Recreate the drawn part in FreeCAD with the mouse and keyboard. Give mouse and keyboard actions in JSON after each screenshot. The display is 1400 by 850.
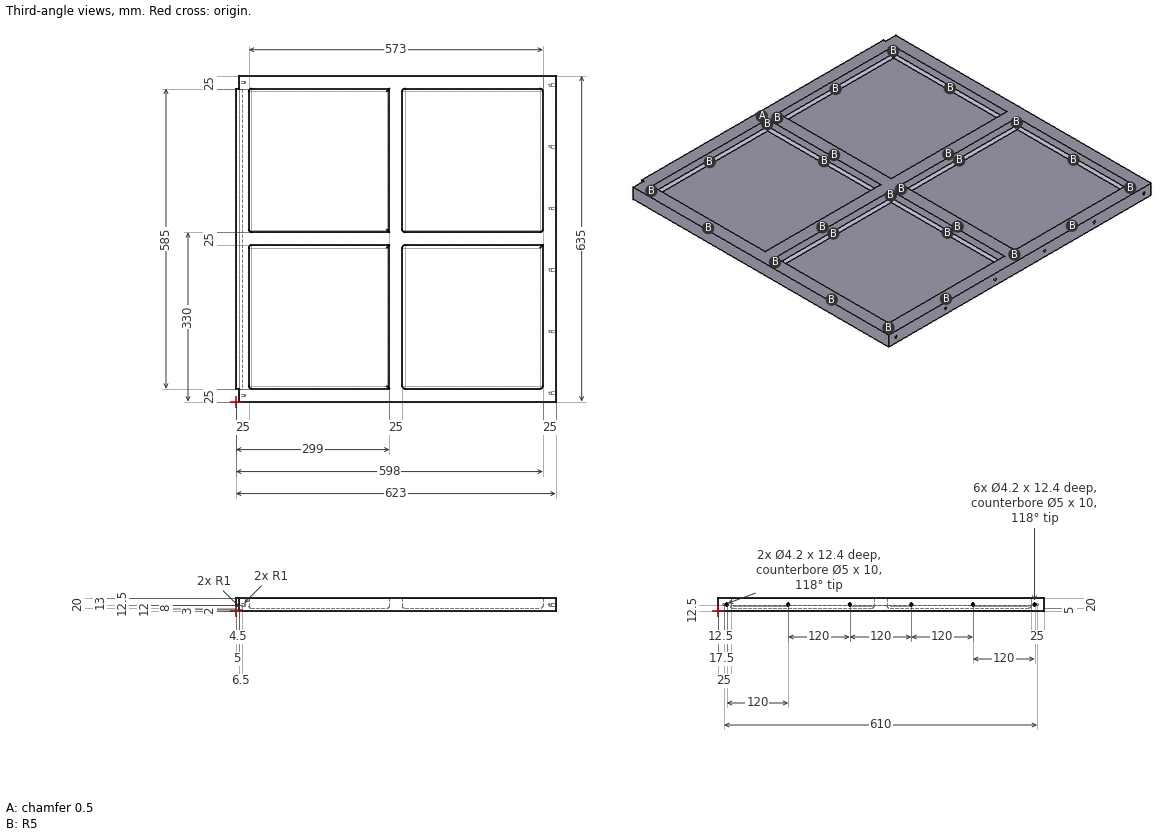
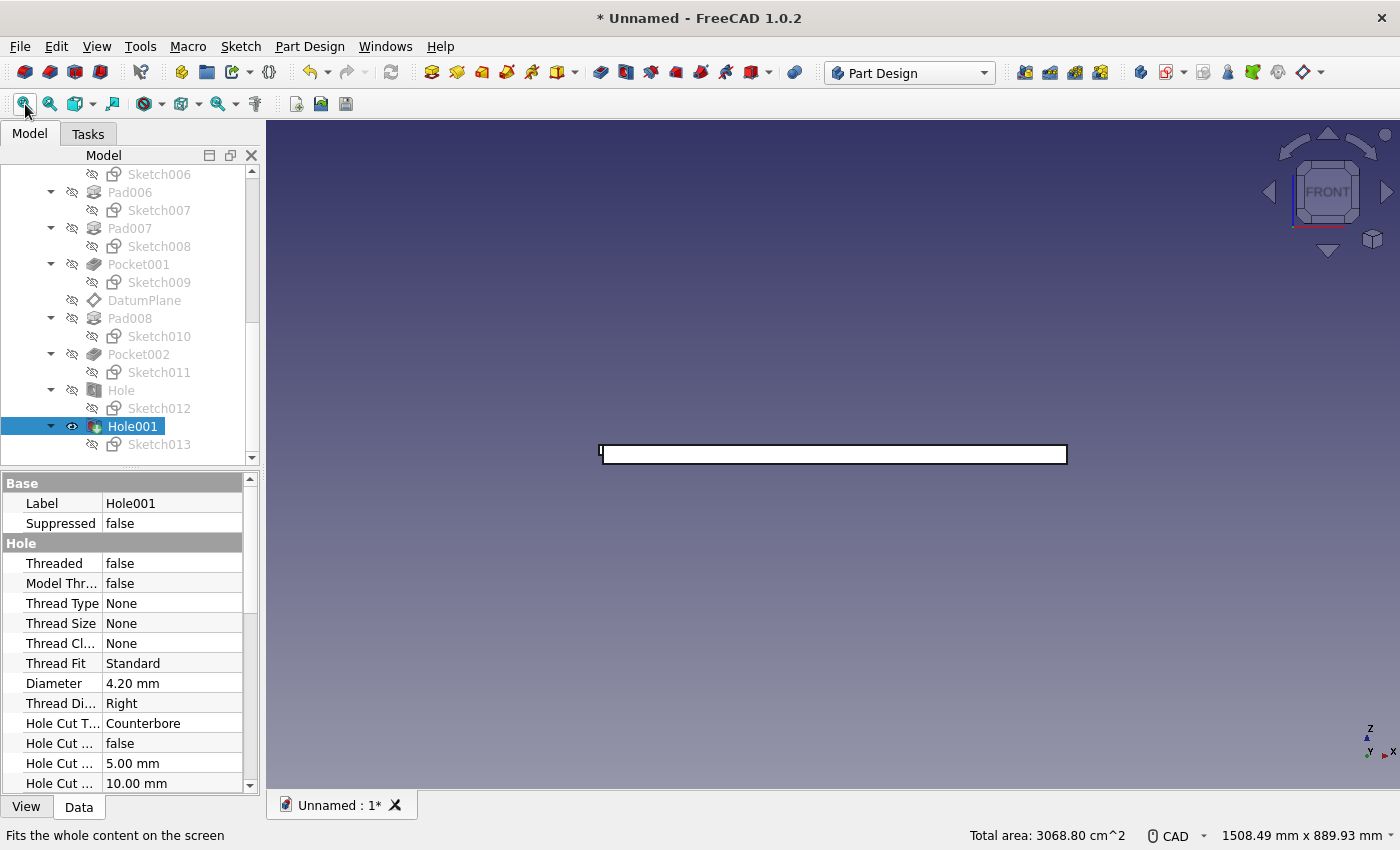
{"action": "left_click", "coordinate": [25, 104]}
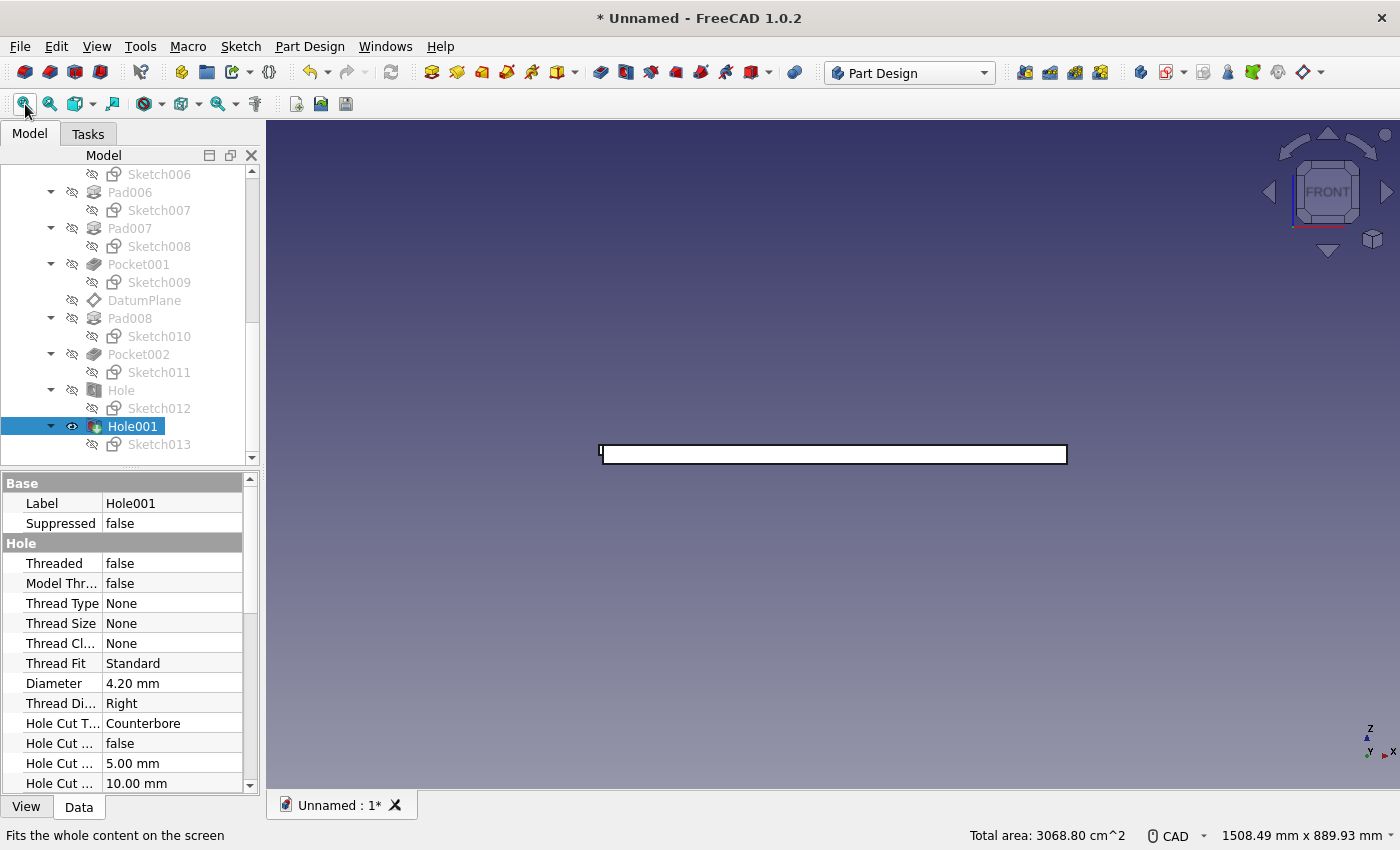
{"action": "scroll", "coordinate": [1048, 452], "scroll_direction": "up", "scroll_amount": 5}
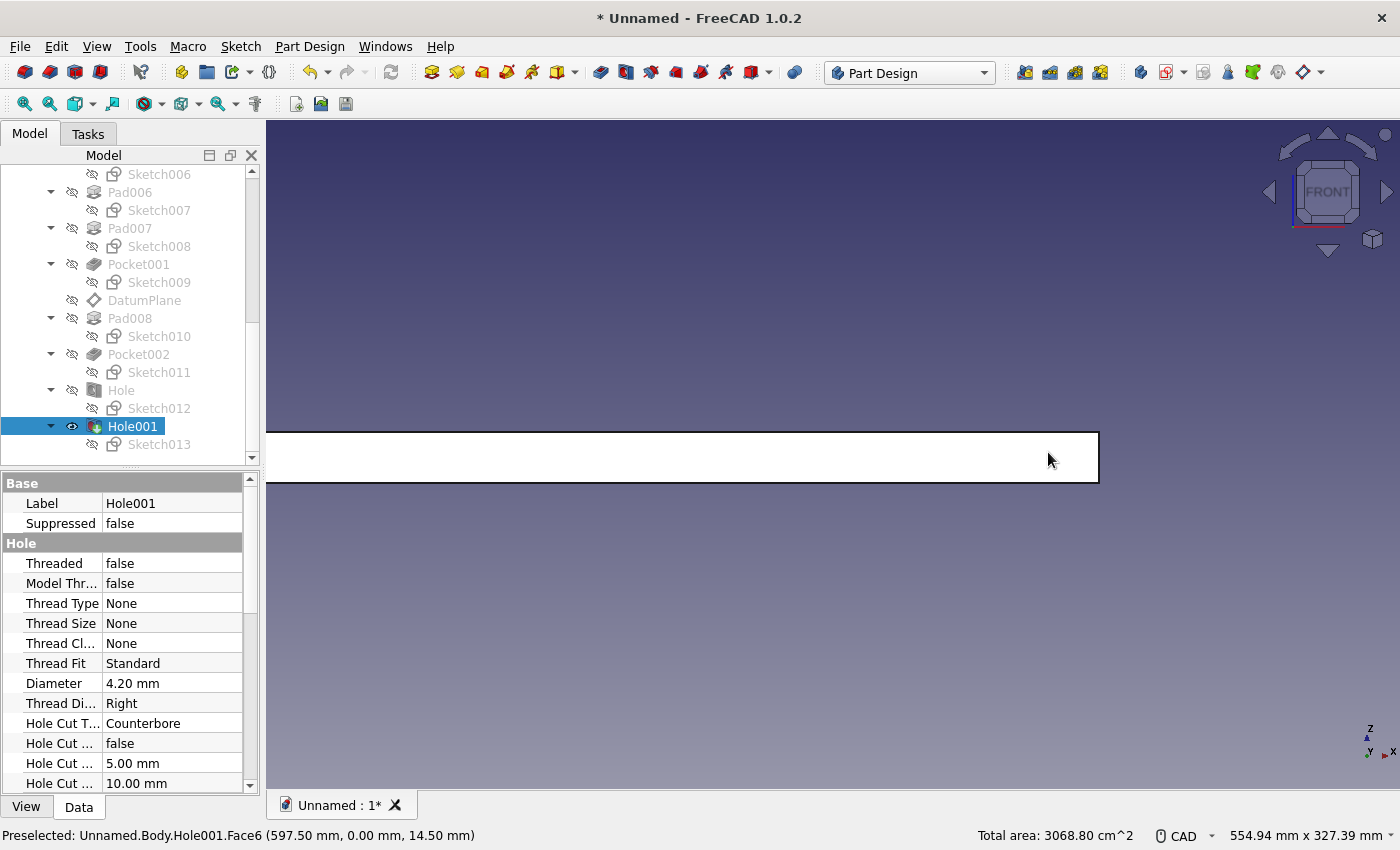
{"action": "left_click", "coordinate": [25, 104]}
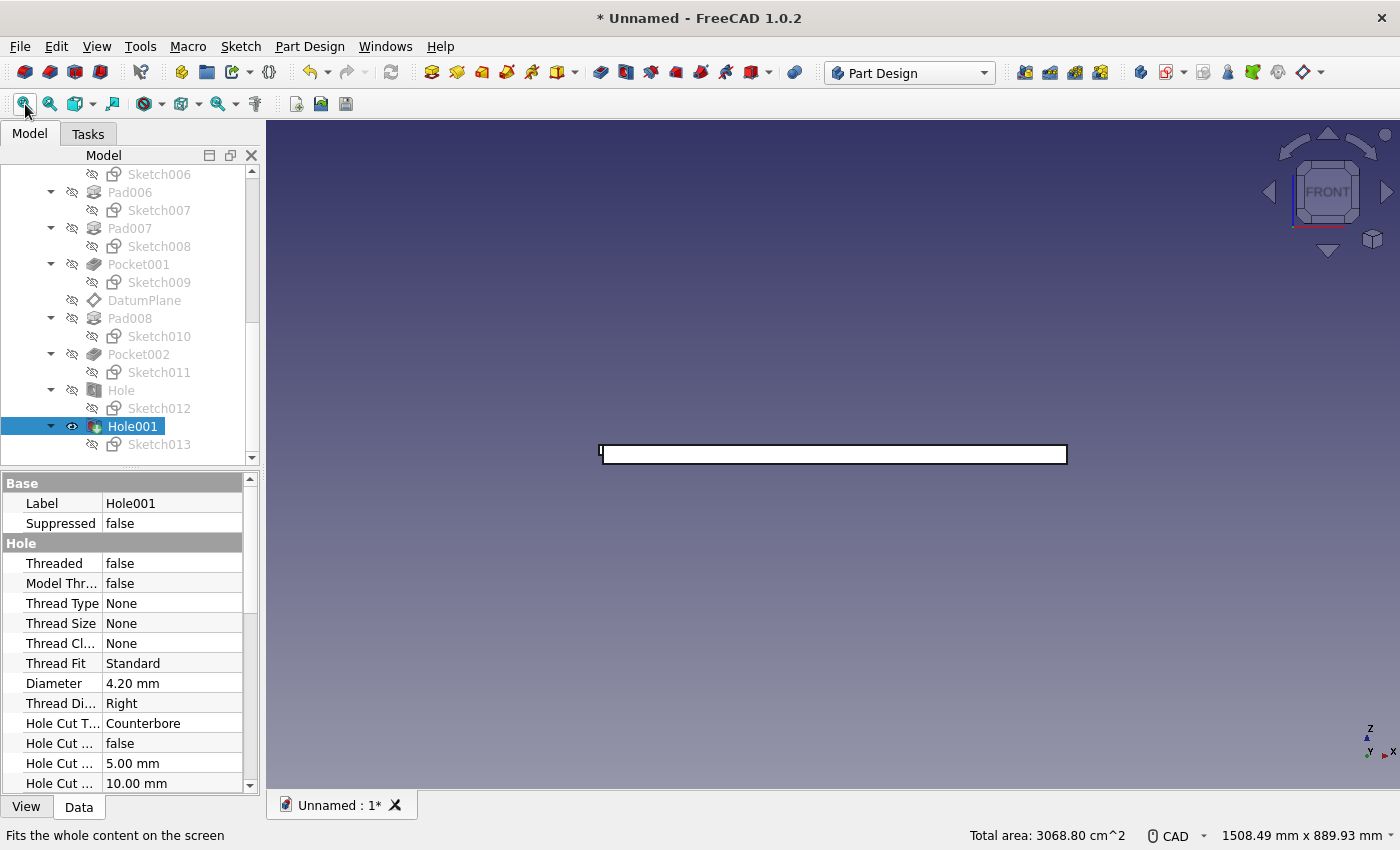
{"action": "key", "text": "3"}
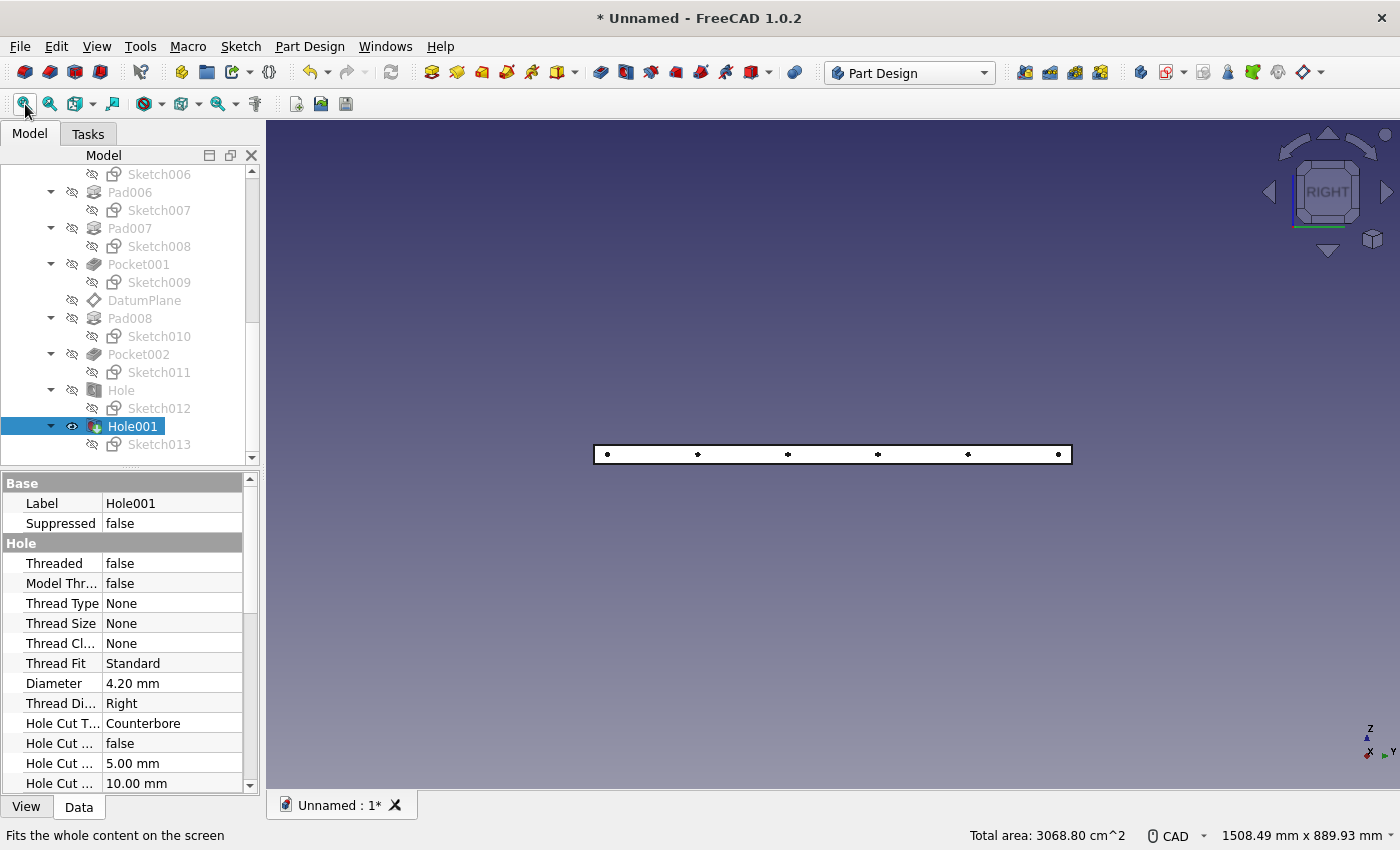
{"action": "left_click", "coordinate": [25, 104]}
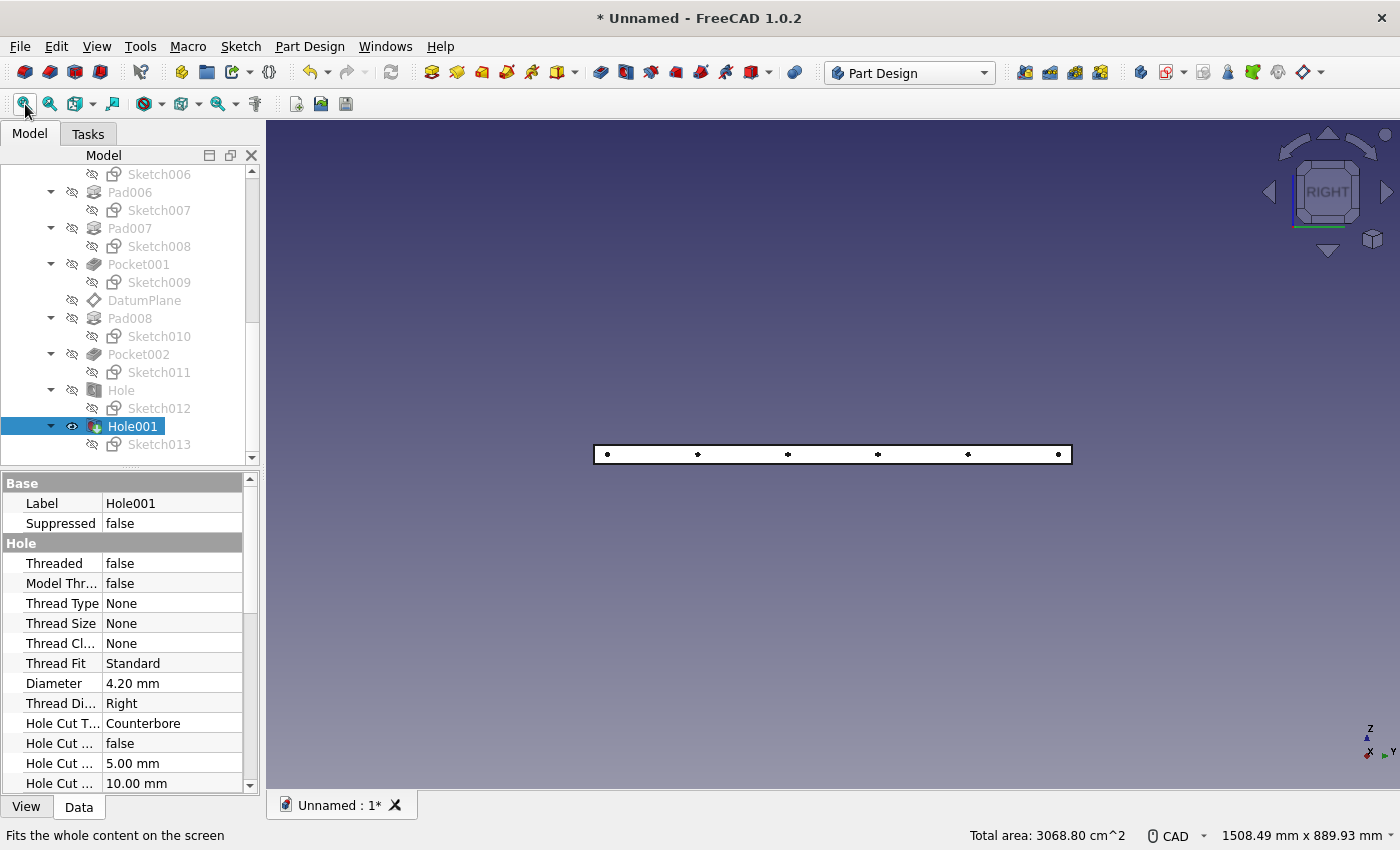
{"action": "scroll", "coordinate": [613, 452], "scroll_direction": "up", "scroll_amount": 5}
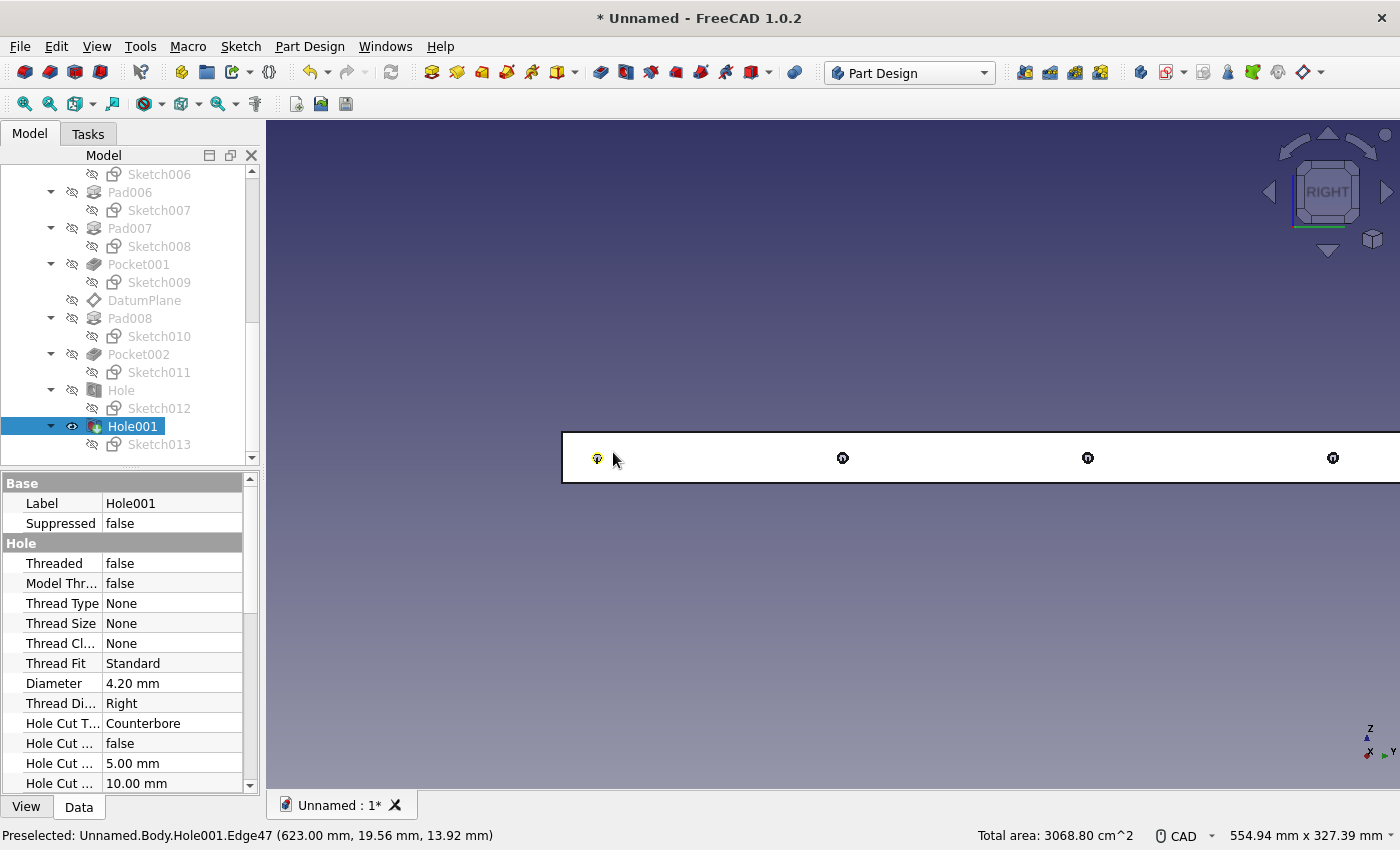
{"action": "left_click", "coordinate": [25, 104]}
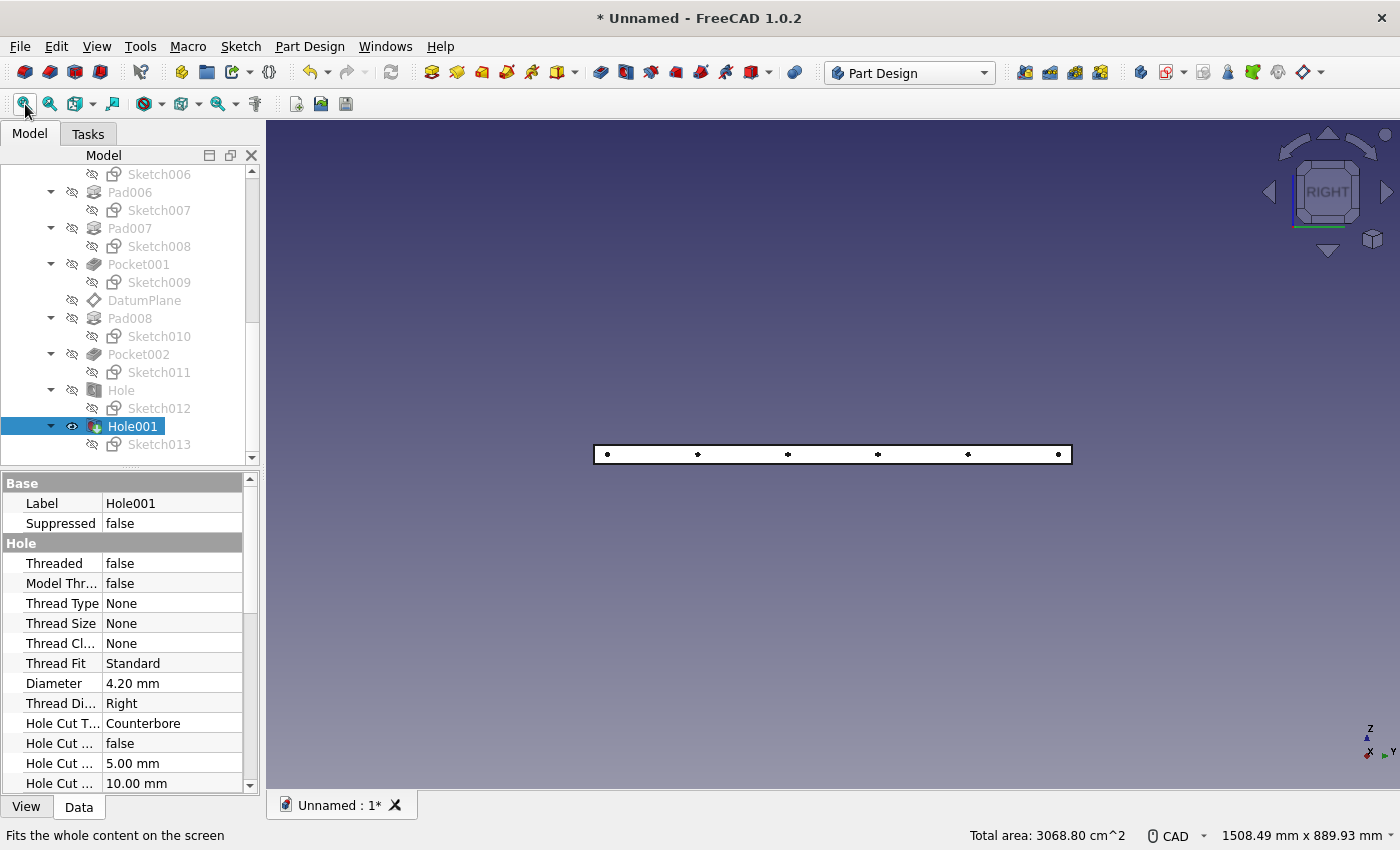
{"action": "key", "text": "5"}